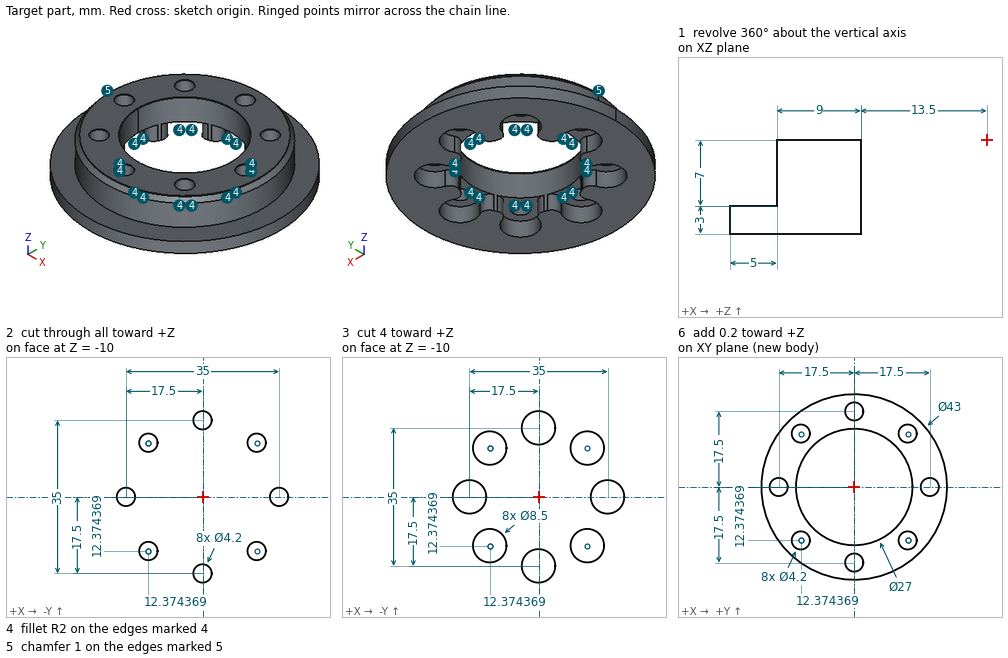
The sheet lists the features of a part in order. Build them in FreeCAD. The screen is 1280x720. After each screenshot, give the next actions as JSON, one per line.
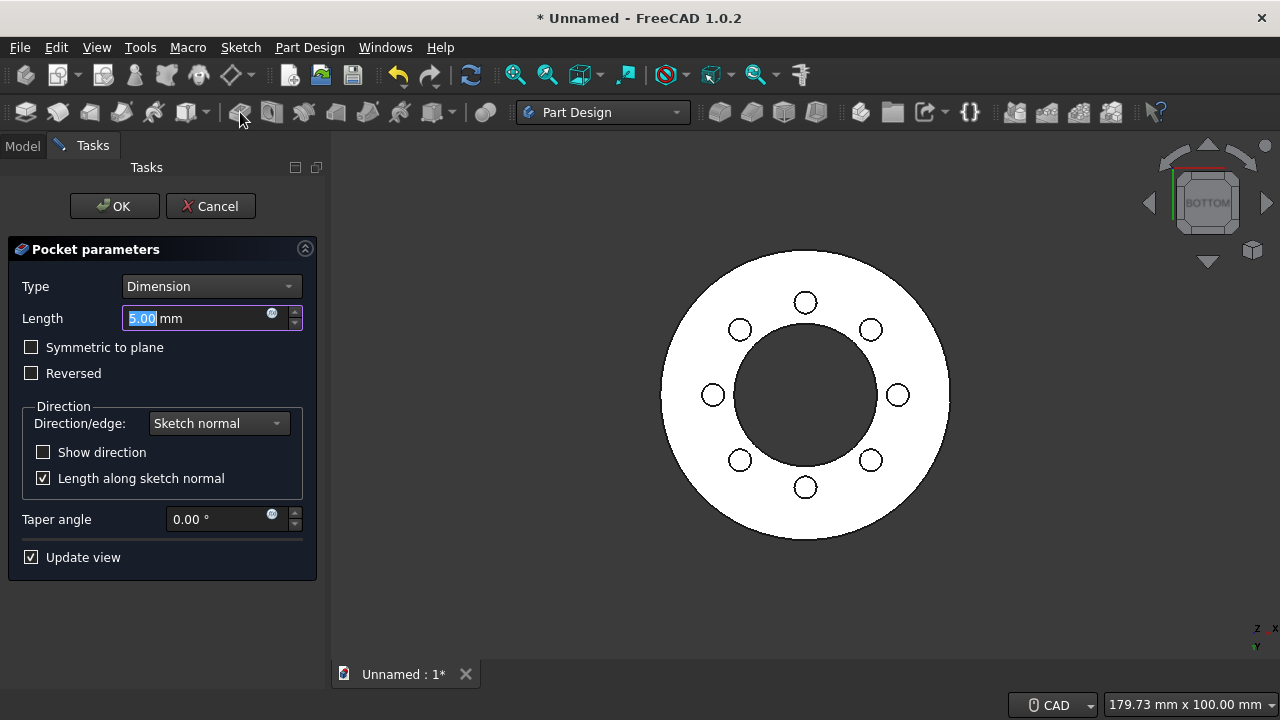
{"action": "left_click", "coordinate": [212, 286]}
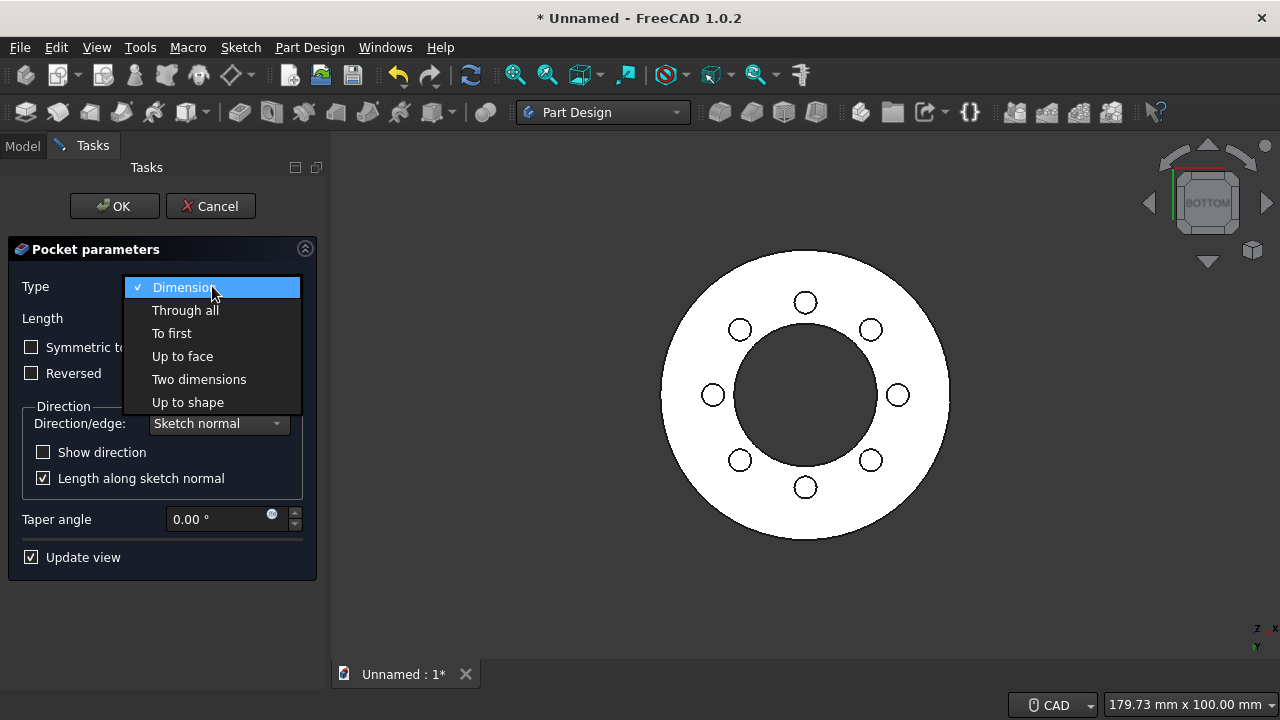
{"action": "left_click", "coordinate": [212, 310]}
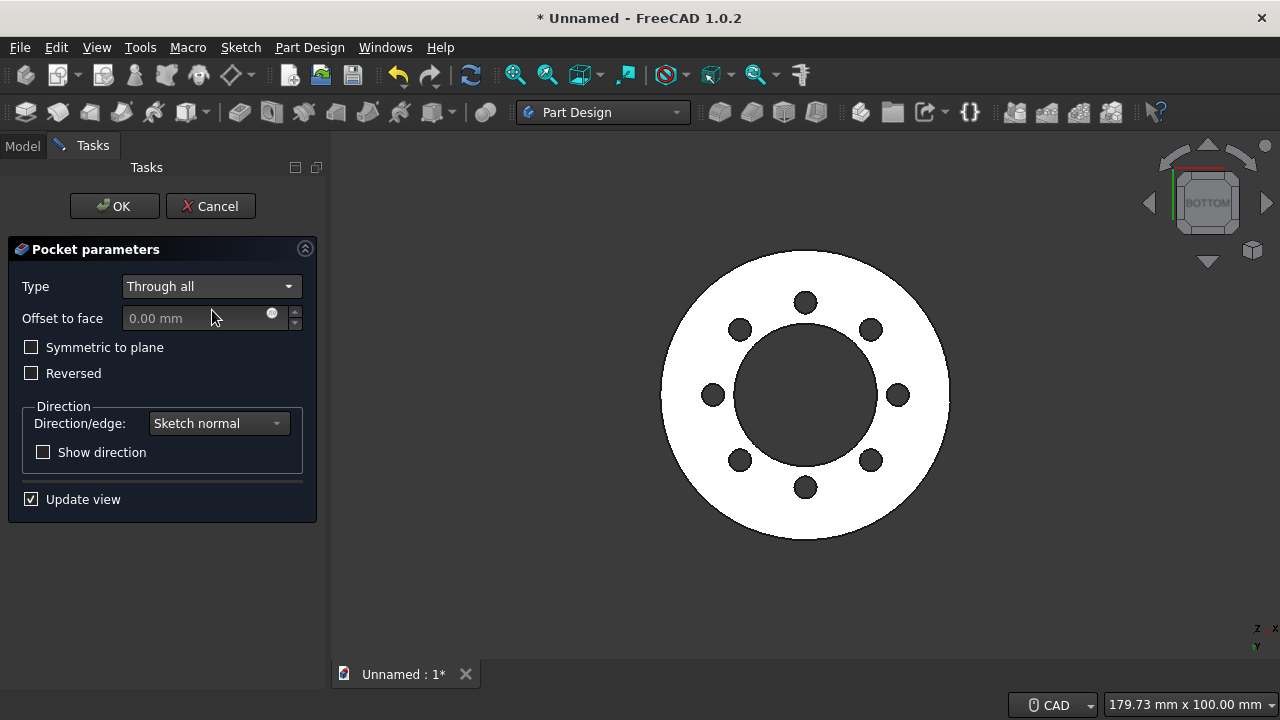
{"action": "left_click", "coordinate": [115, 206]}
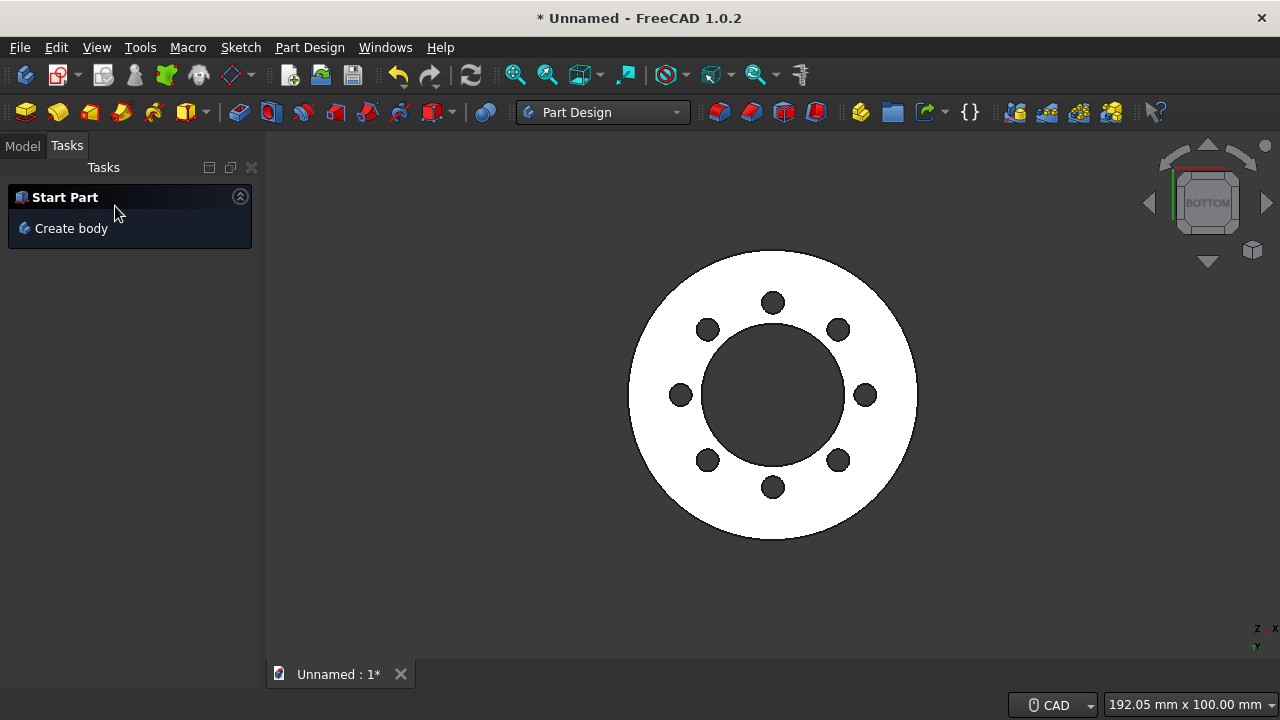
{"action": "left_click", "coordinate": [773, 270]}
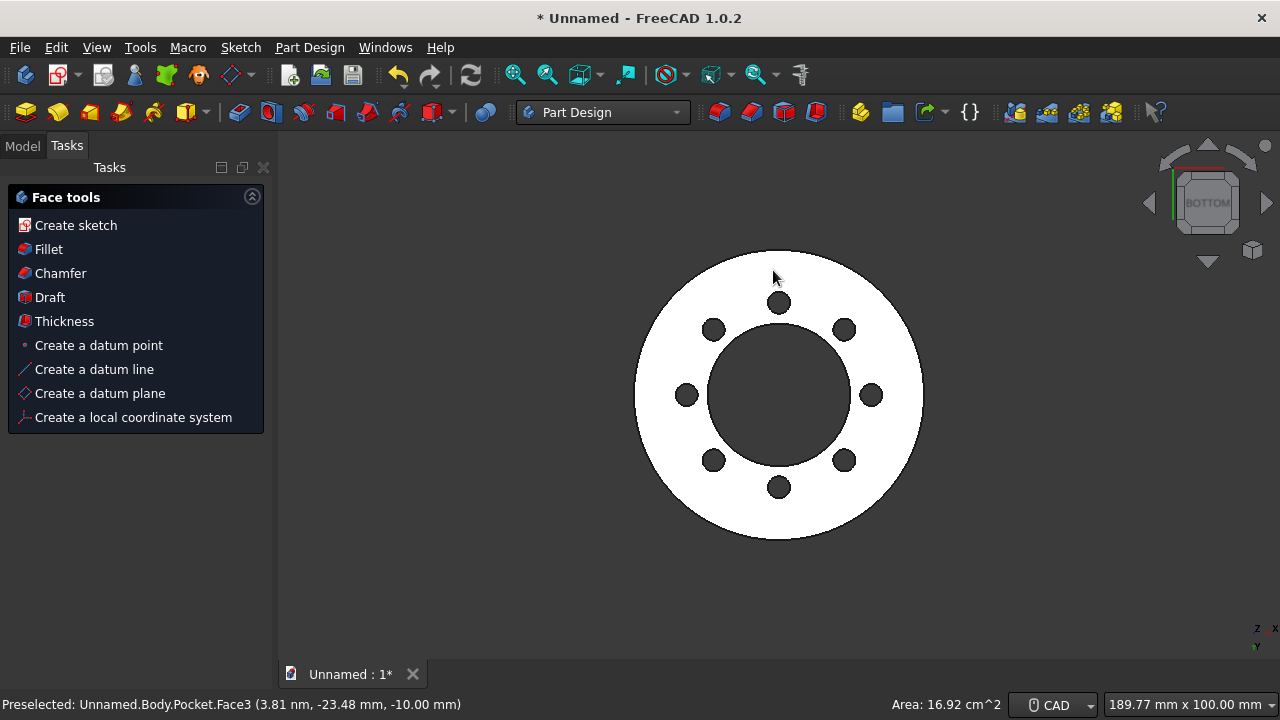
{"action": "left_click", "coordinate": [58, 76]}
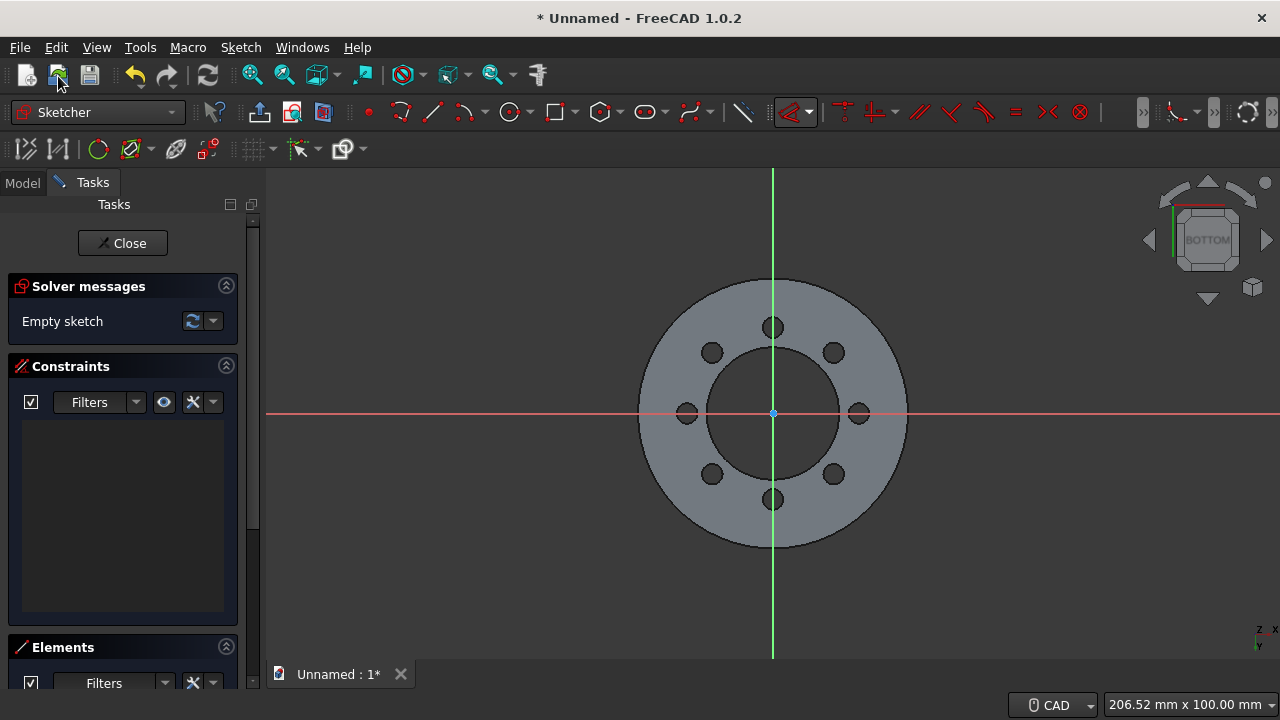
{"action": "scroll", "coordinate": [912, 414], "scroll_direction": "up", "scroll_amount": 2}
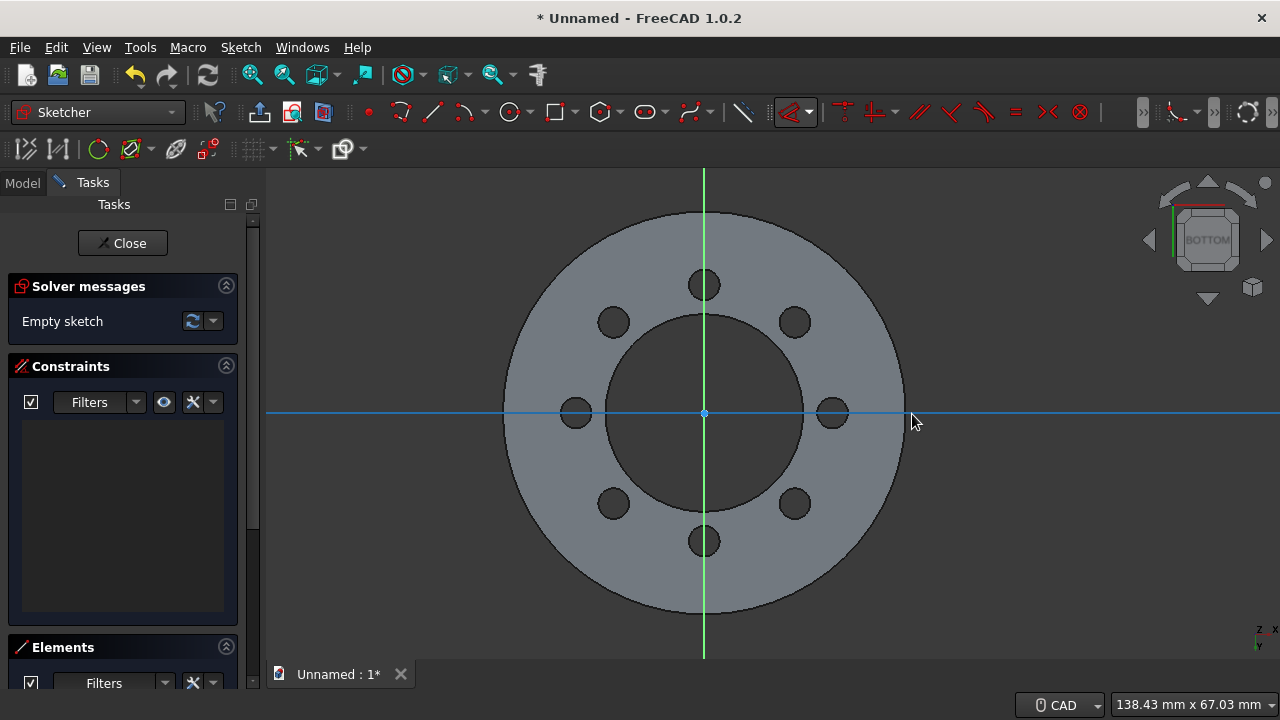
{"action": "left_click", "coordinate": [510, 112]}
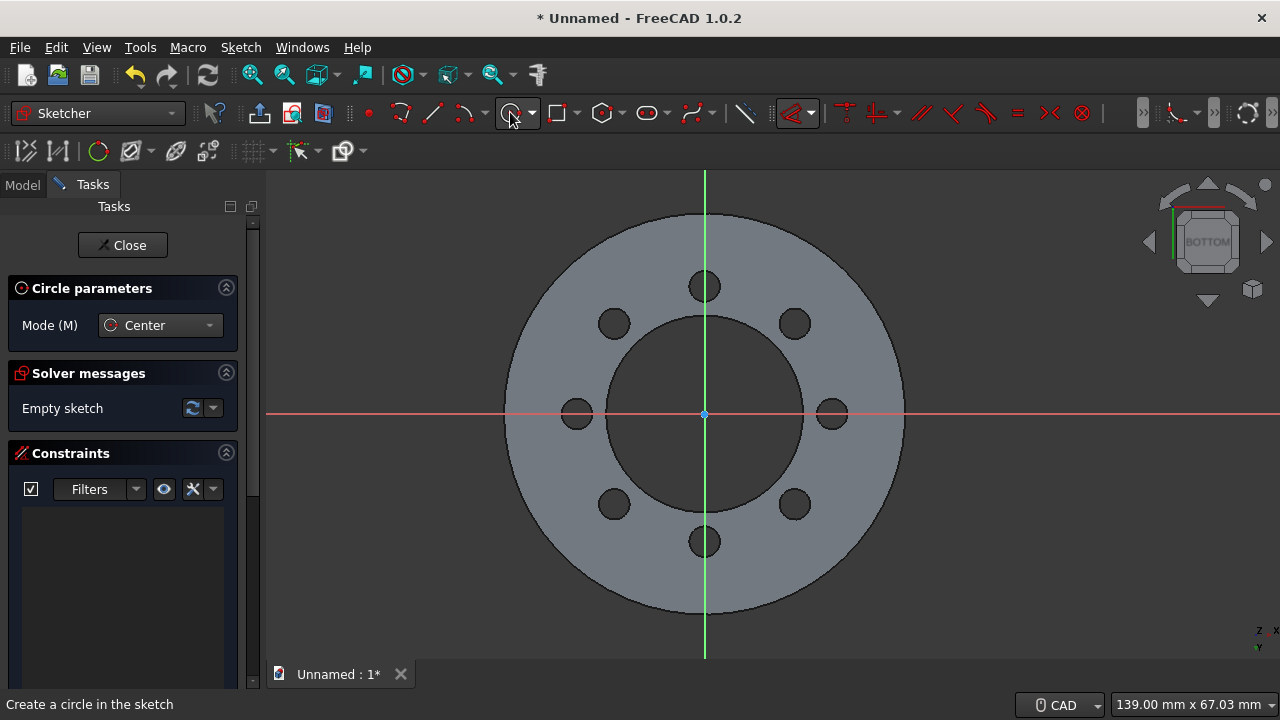
{"action": "left_click", "coordinate": [705, 542]}
{"action": "mouse_move", "coordinate": [727, 520]}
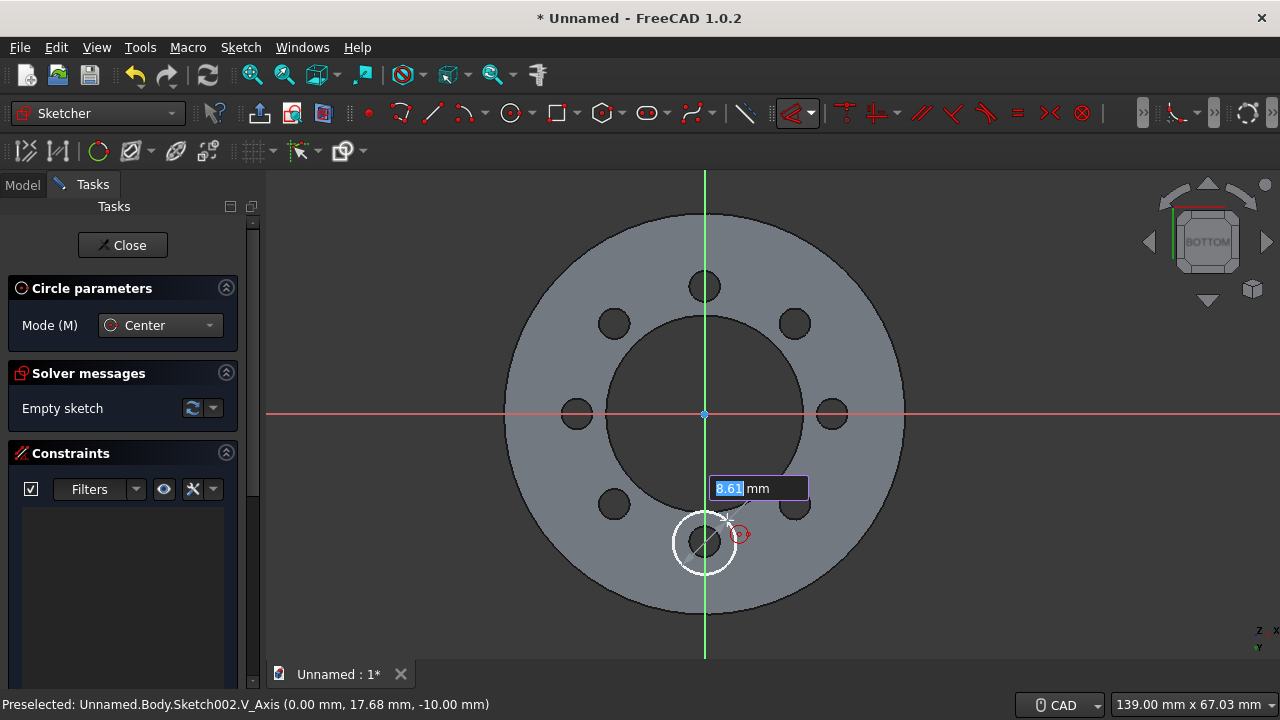
{"action": "type", "text": "8.5"}
{"action": "key", "text": "Return"}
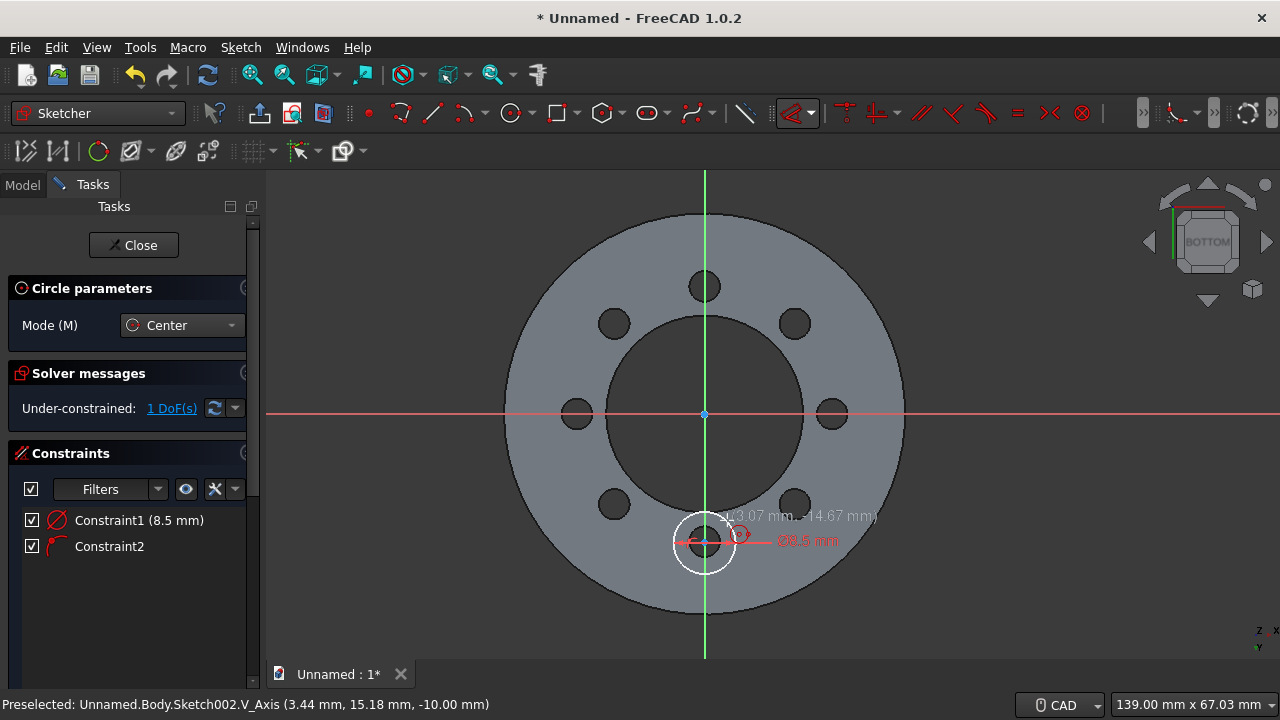
{"action": "left_click", "coordinate": [614, 504]}
{"action": "mouse_move", "coordinate": [636, 482]}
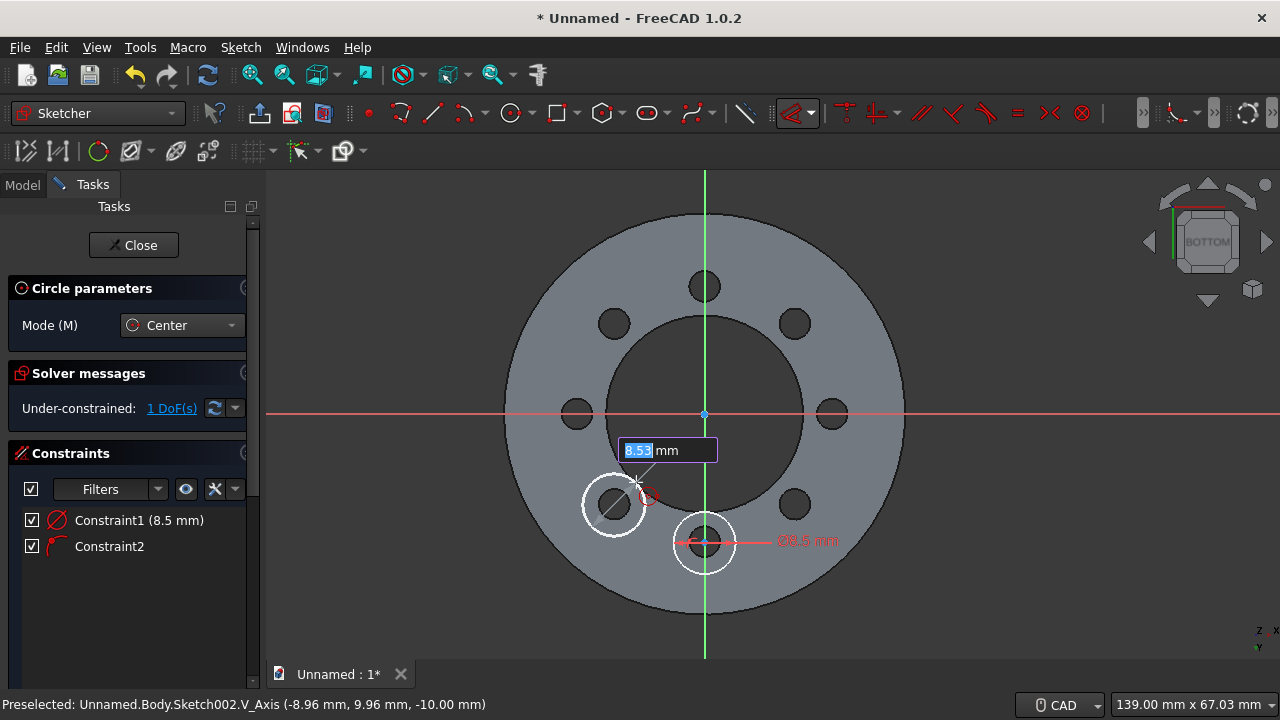
{"action": "type", "text": "8.5"}
{"action": "key", "text": "Return"}